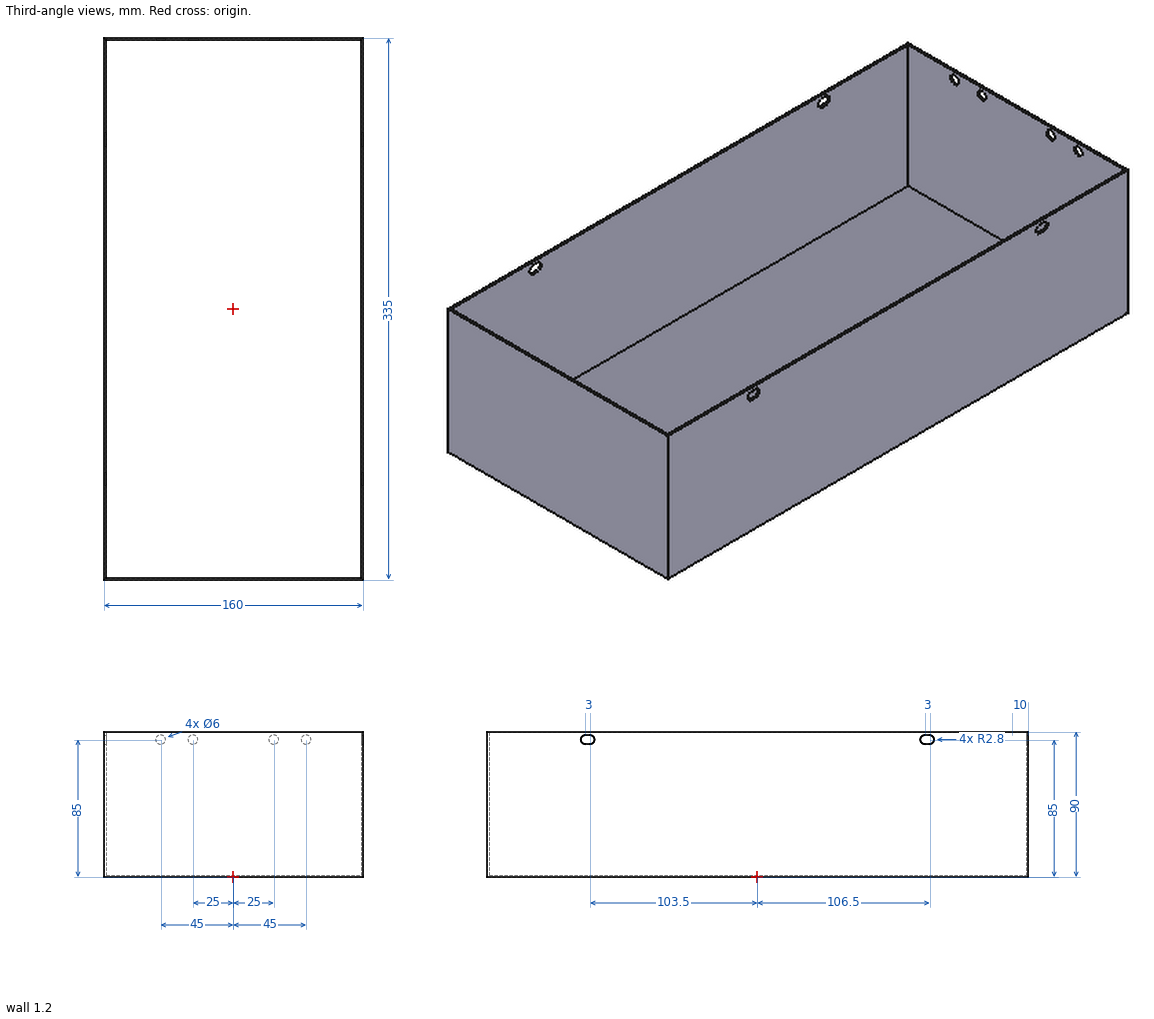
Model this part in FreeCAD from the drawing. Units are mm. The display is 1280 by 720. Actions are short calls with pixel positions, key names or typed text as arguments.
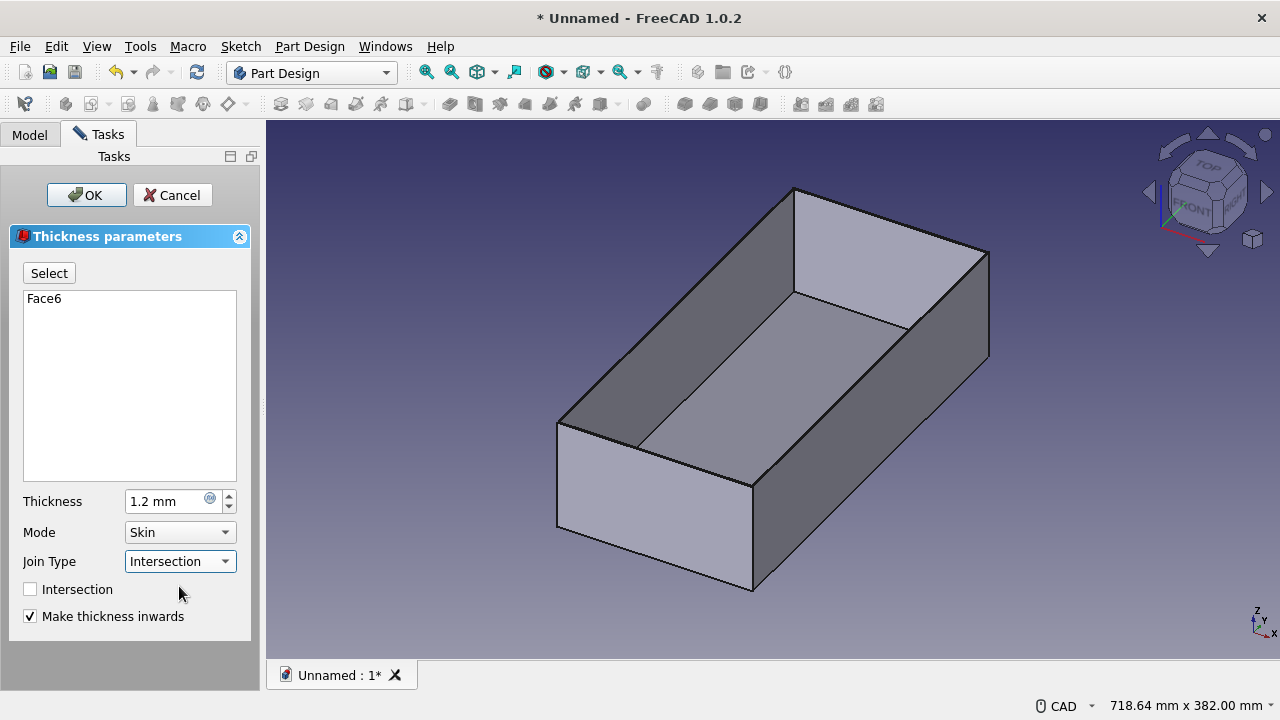
click(87, 195)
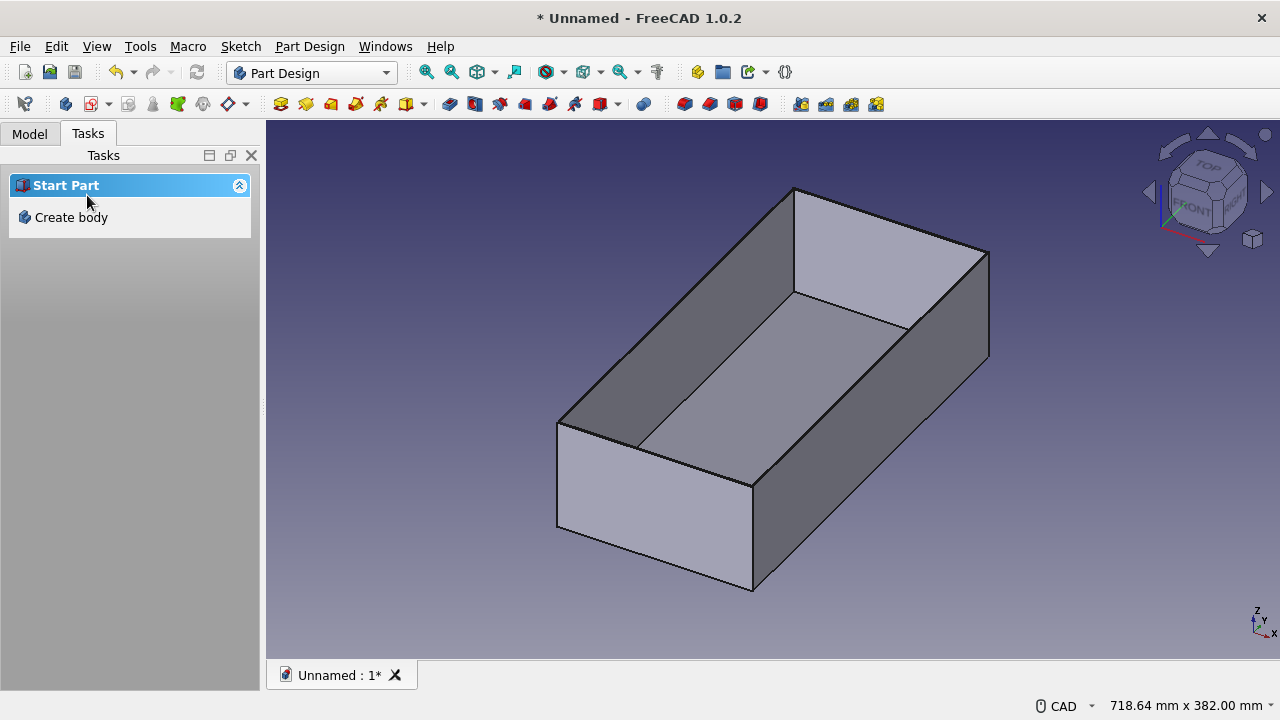
key(4)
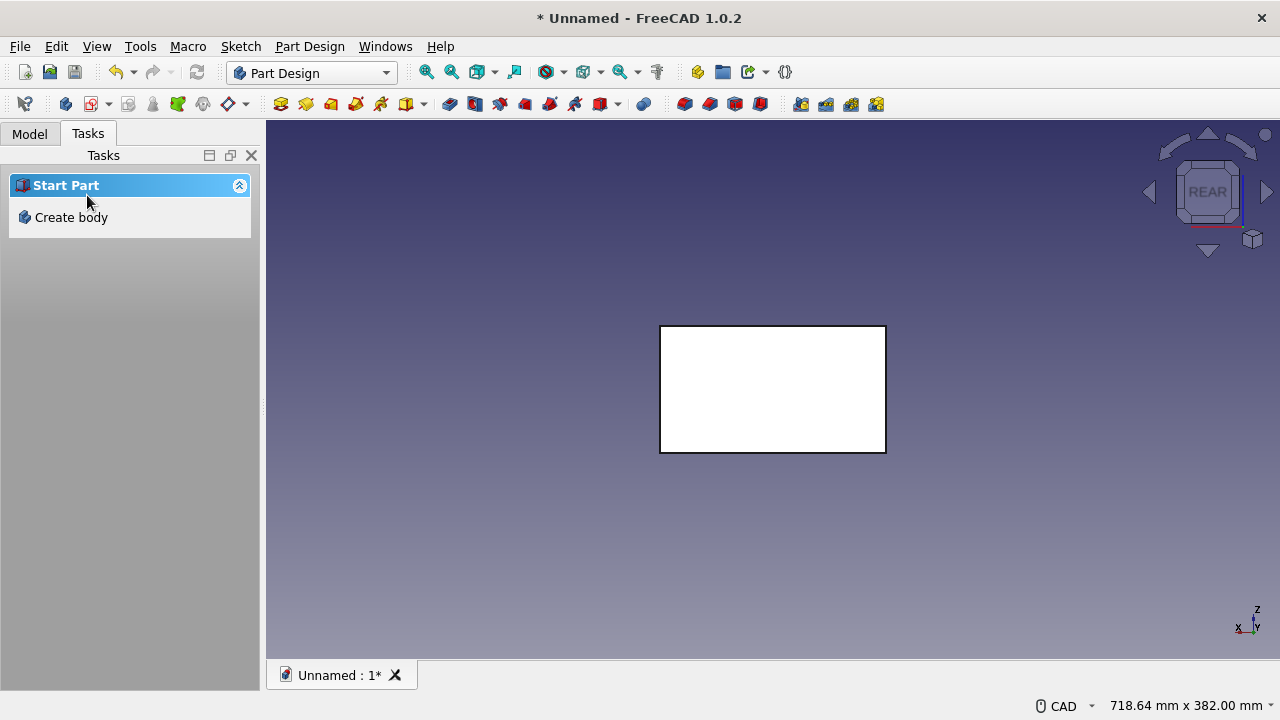
key(v)
key(f)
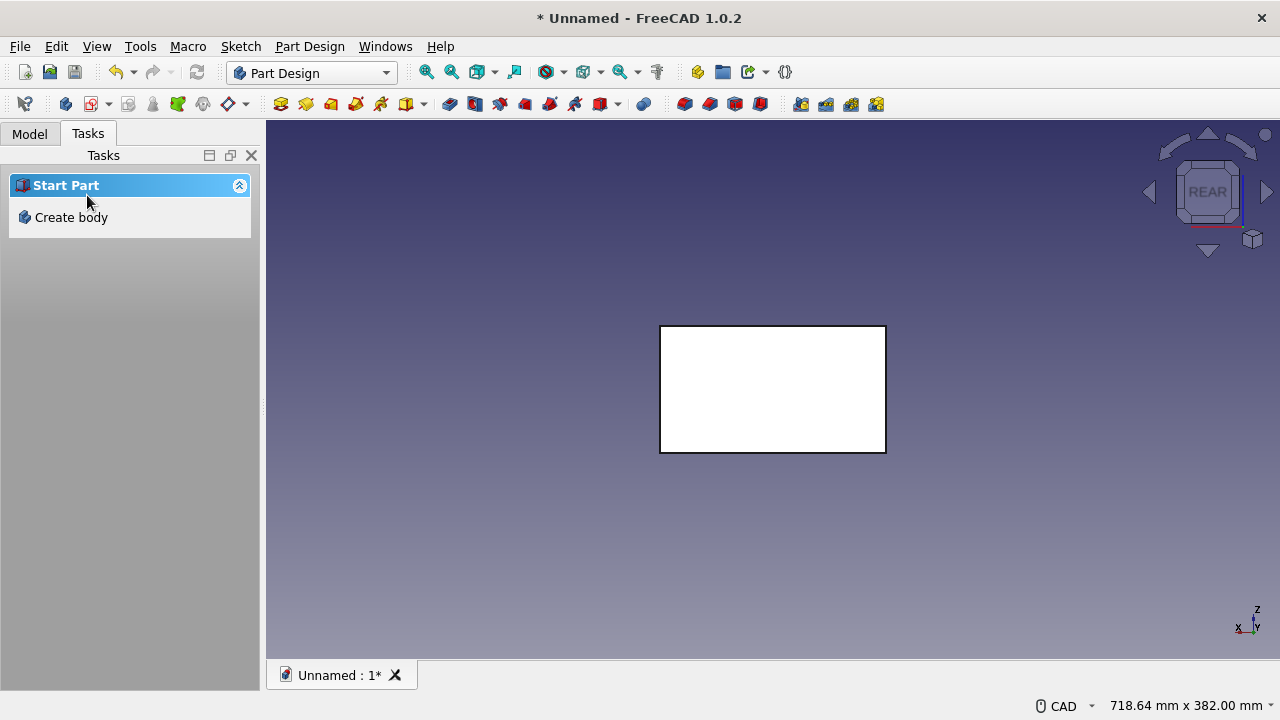
click(741, 389)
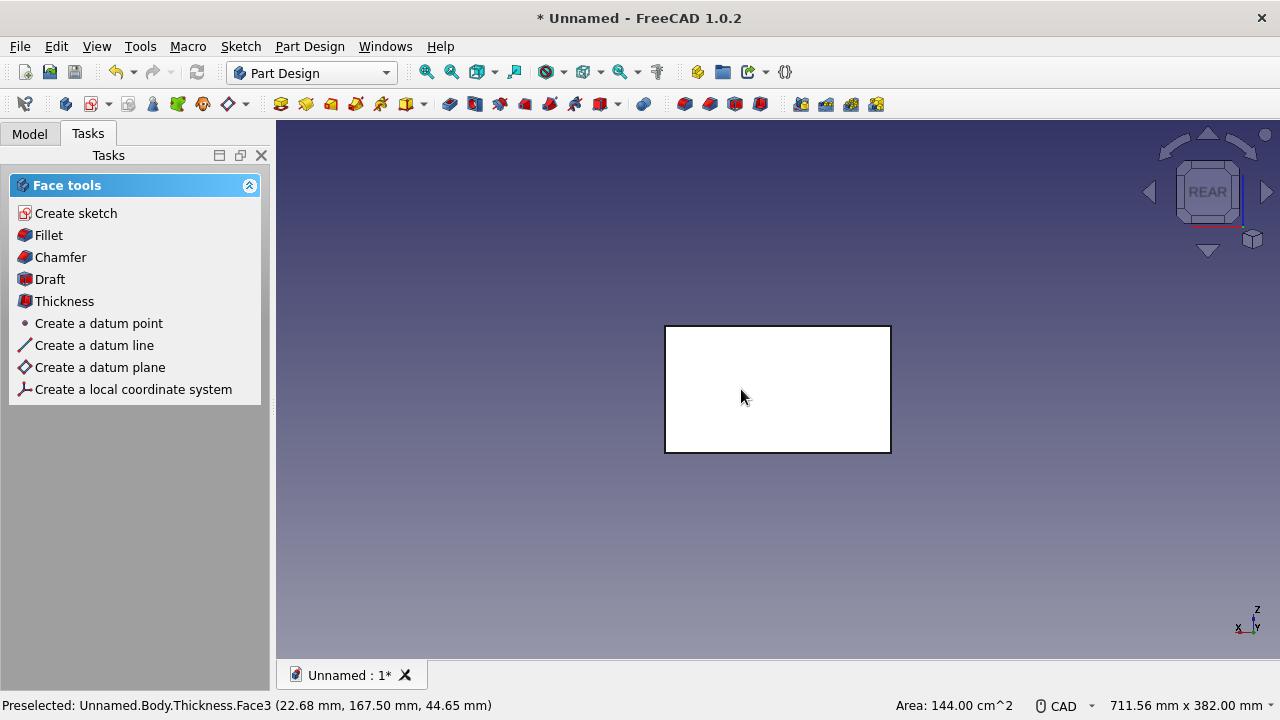
click(90, 104)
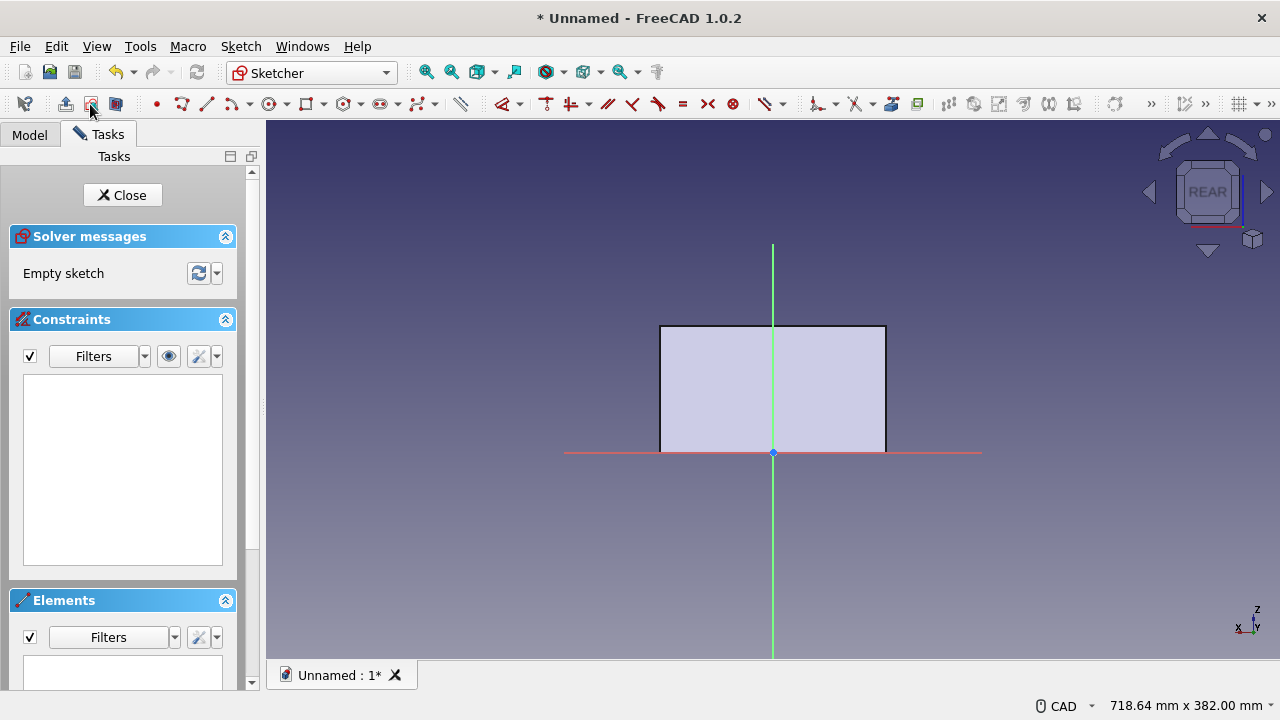
scroll(813, 392, up, 5)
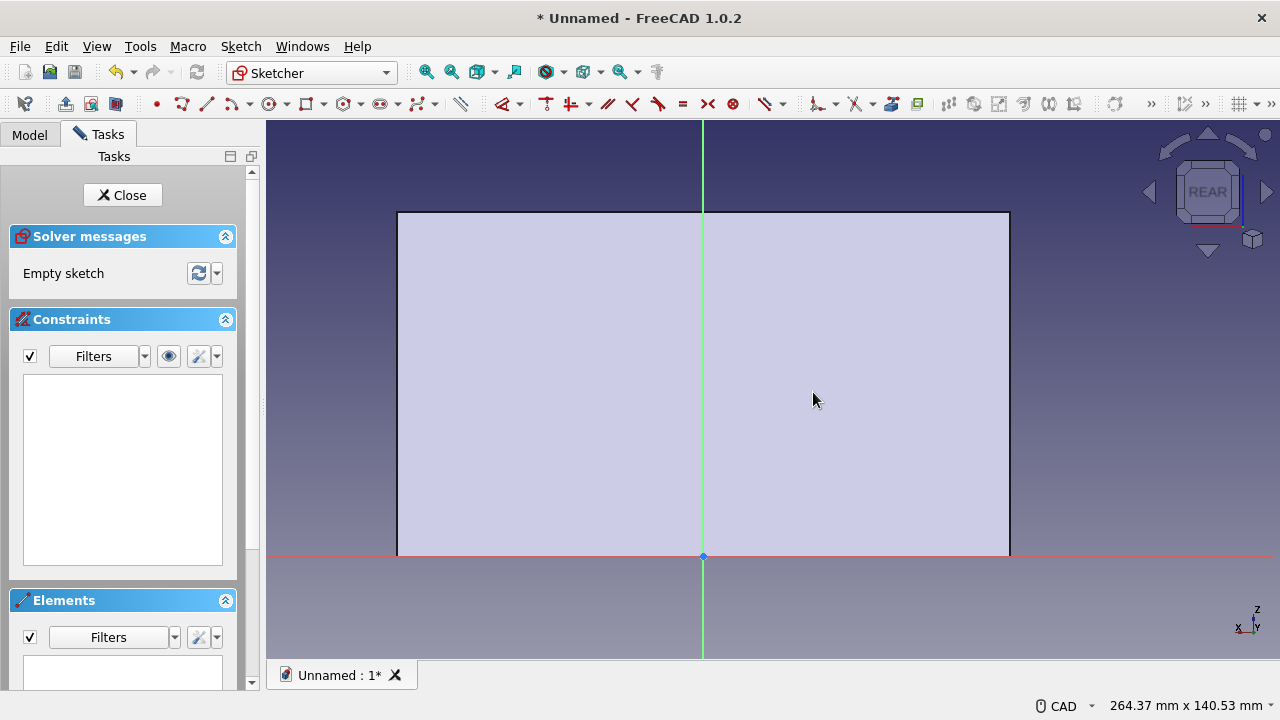
click(268, 104)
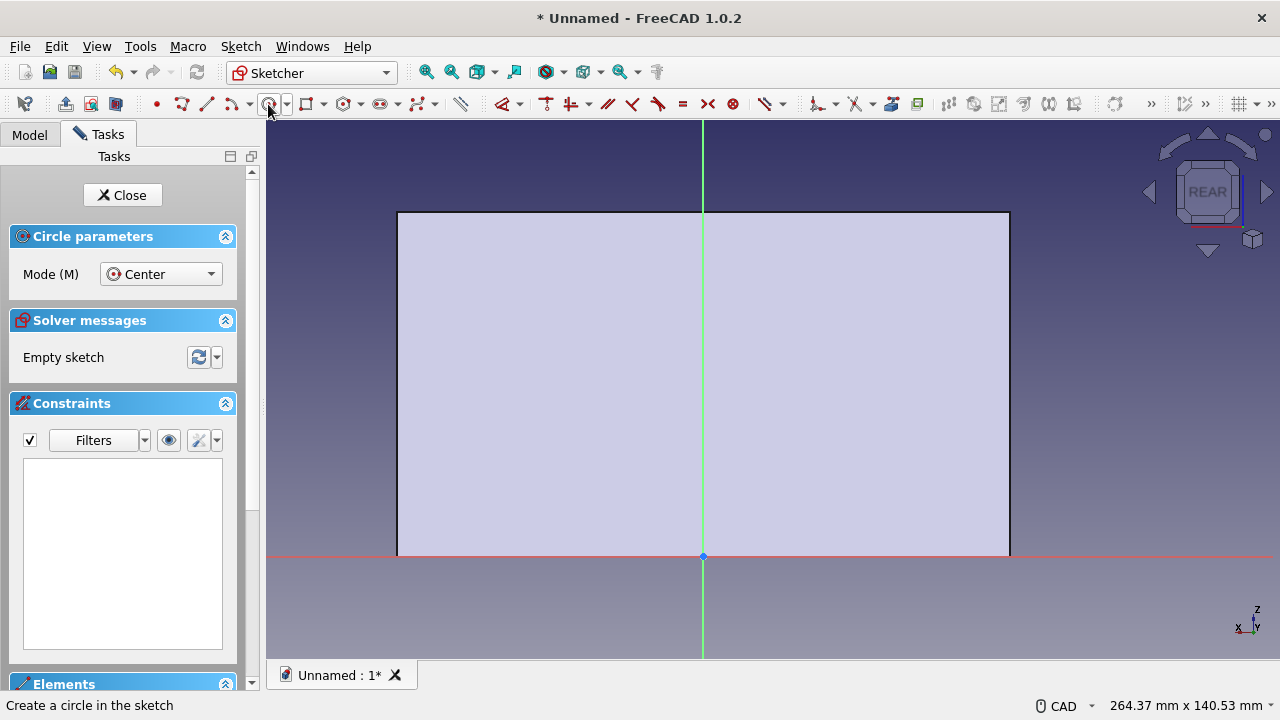
scroll(876, 231, up, 4)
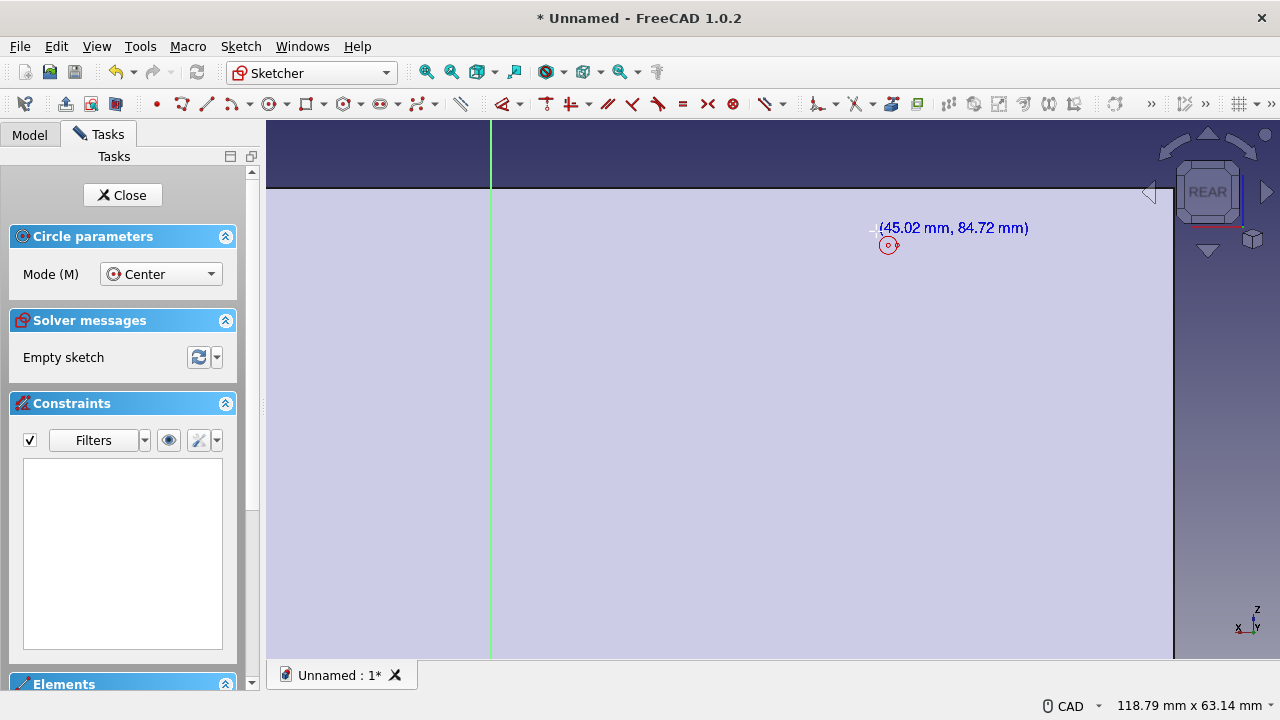
click(875, 231)
click(893, 212)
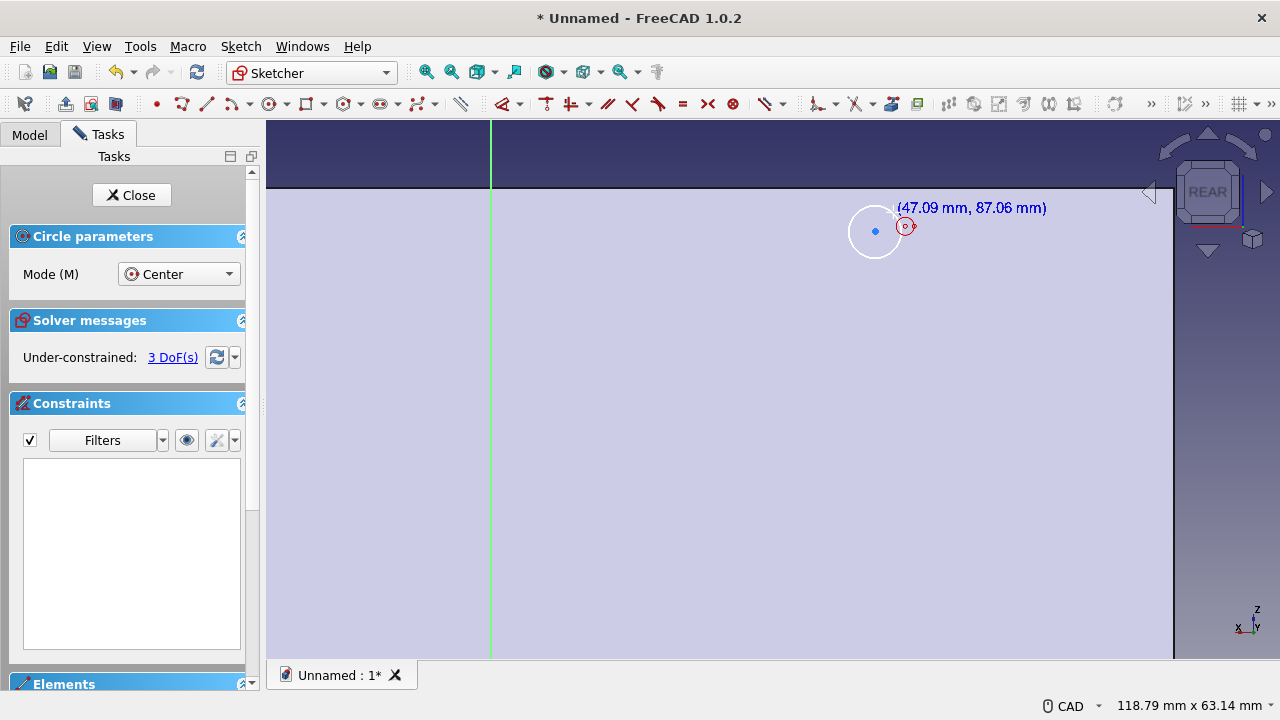
click(704, 231)
click(723, 212)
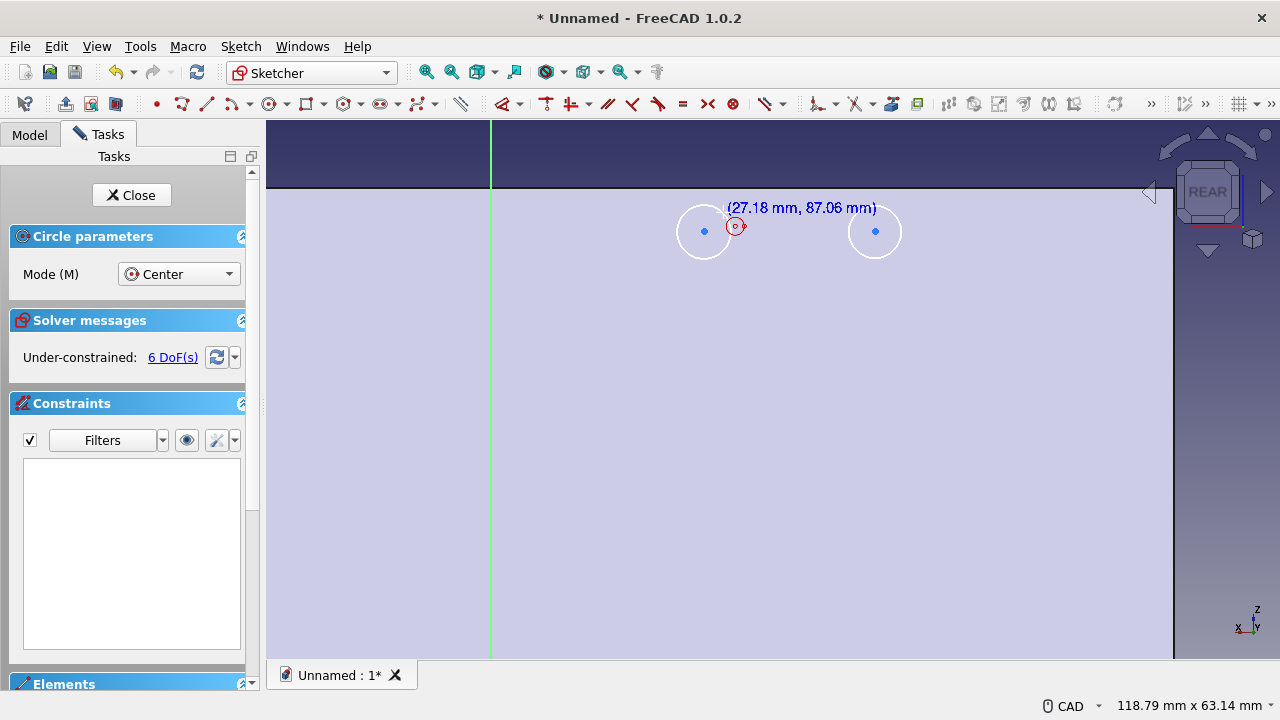
scroll(879, 234, down, 4)